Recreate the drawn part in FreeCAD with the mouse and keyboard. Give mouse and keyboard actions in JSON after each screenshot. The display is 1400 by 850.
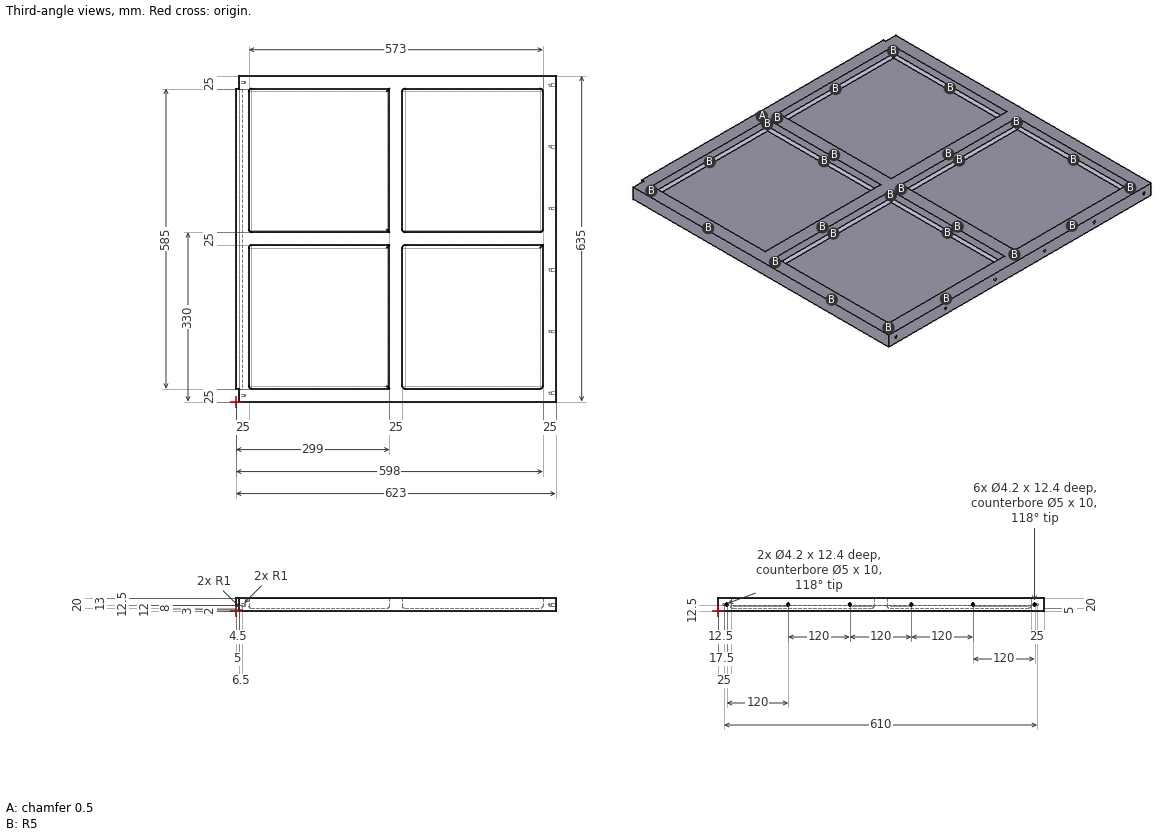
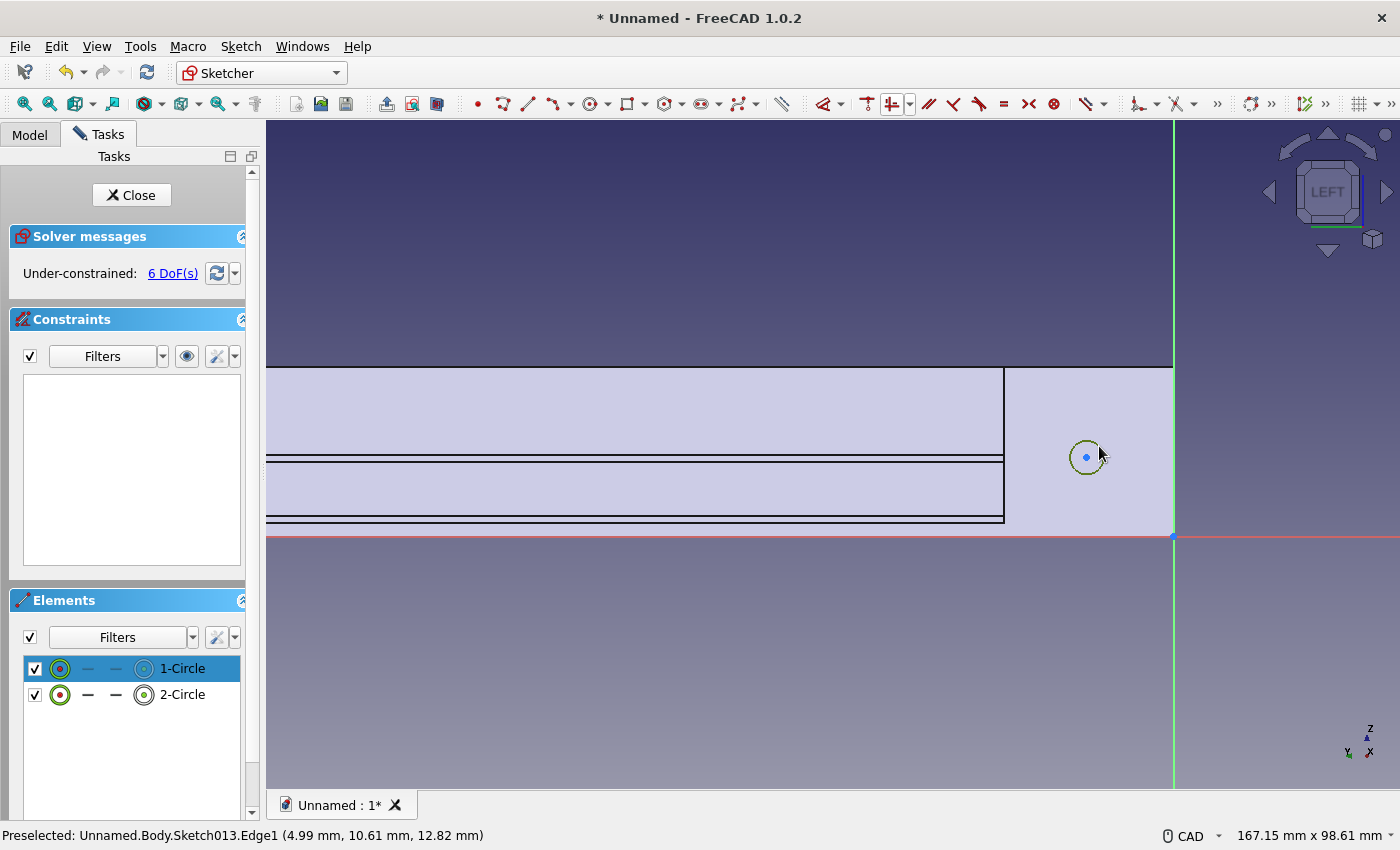
{"action": "scroll", "coordinate": [1103, 448], "scroll_direction": "down", "scroll_amount": 9}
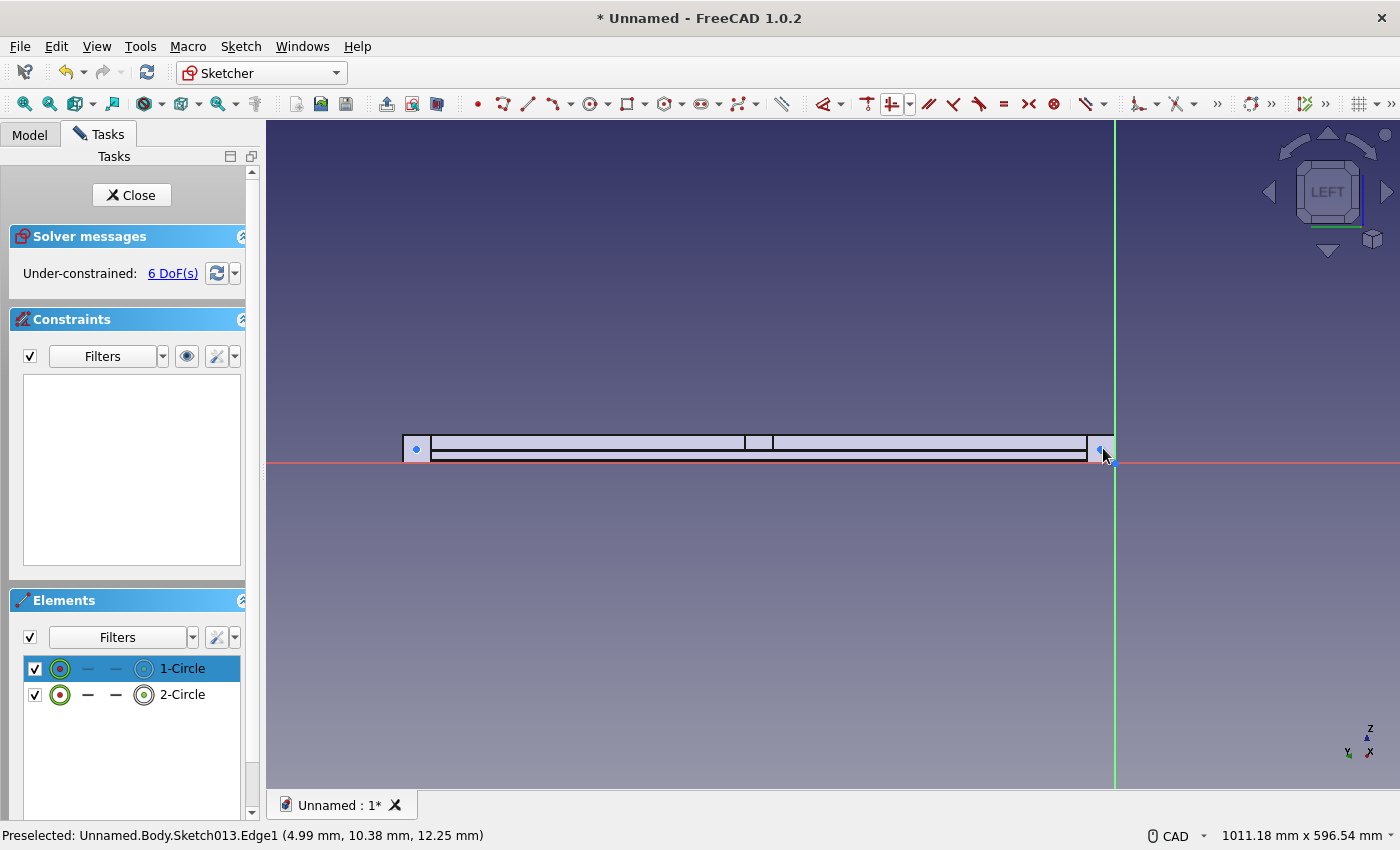
{"action": "scroll", "coordinate": [419, 448], "scroll_direction": "up", "scroll_amount": 8}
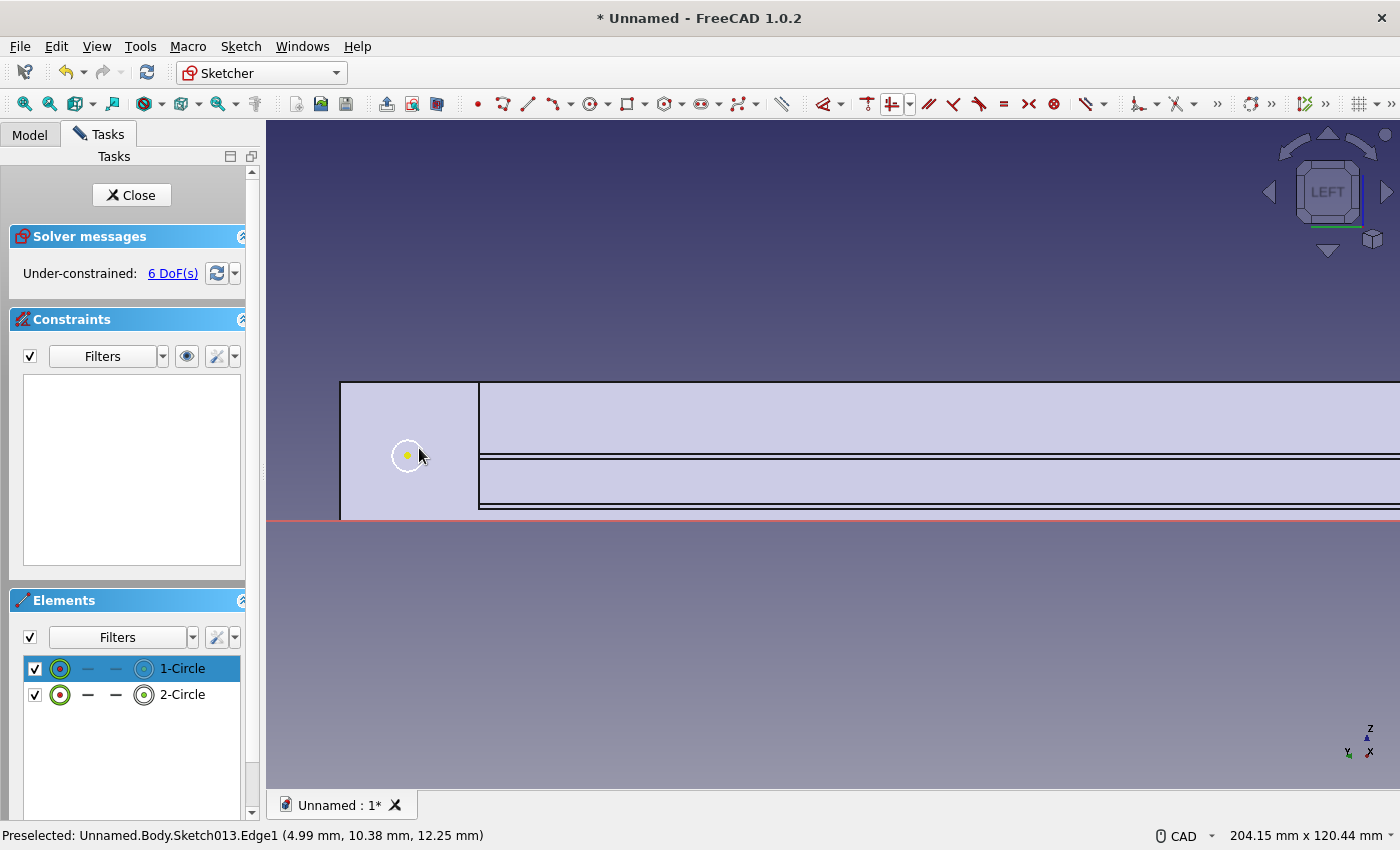
{"action": "left_click", "coordinate": [419, 445]}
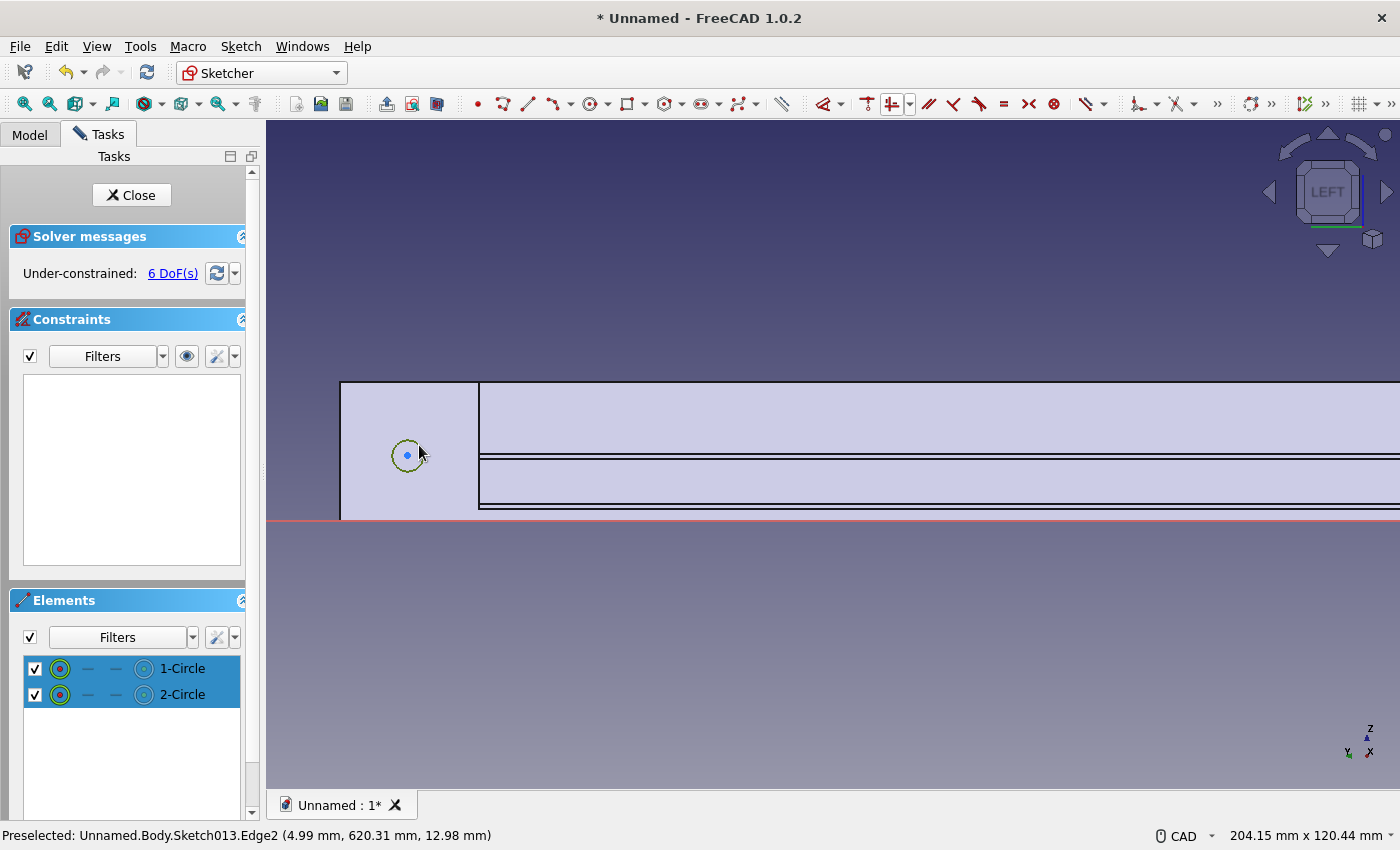
{"action": "left_click", "coordinate": [1004, 104]}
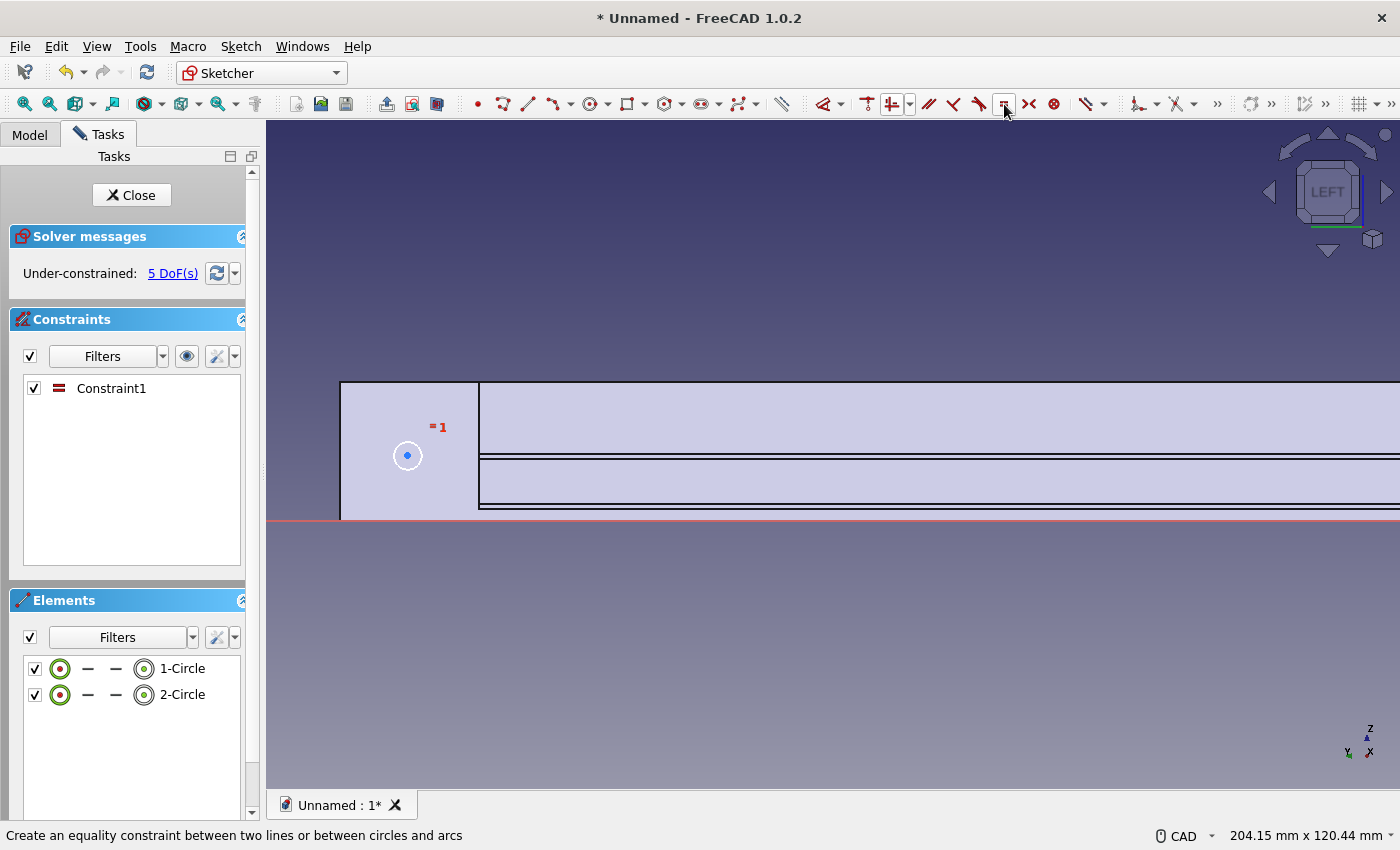
{"action": "left_click", "coordinate": [822, 104]}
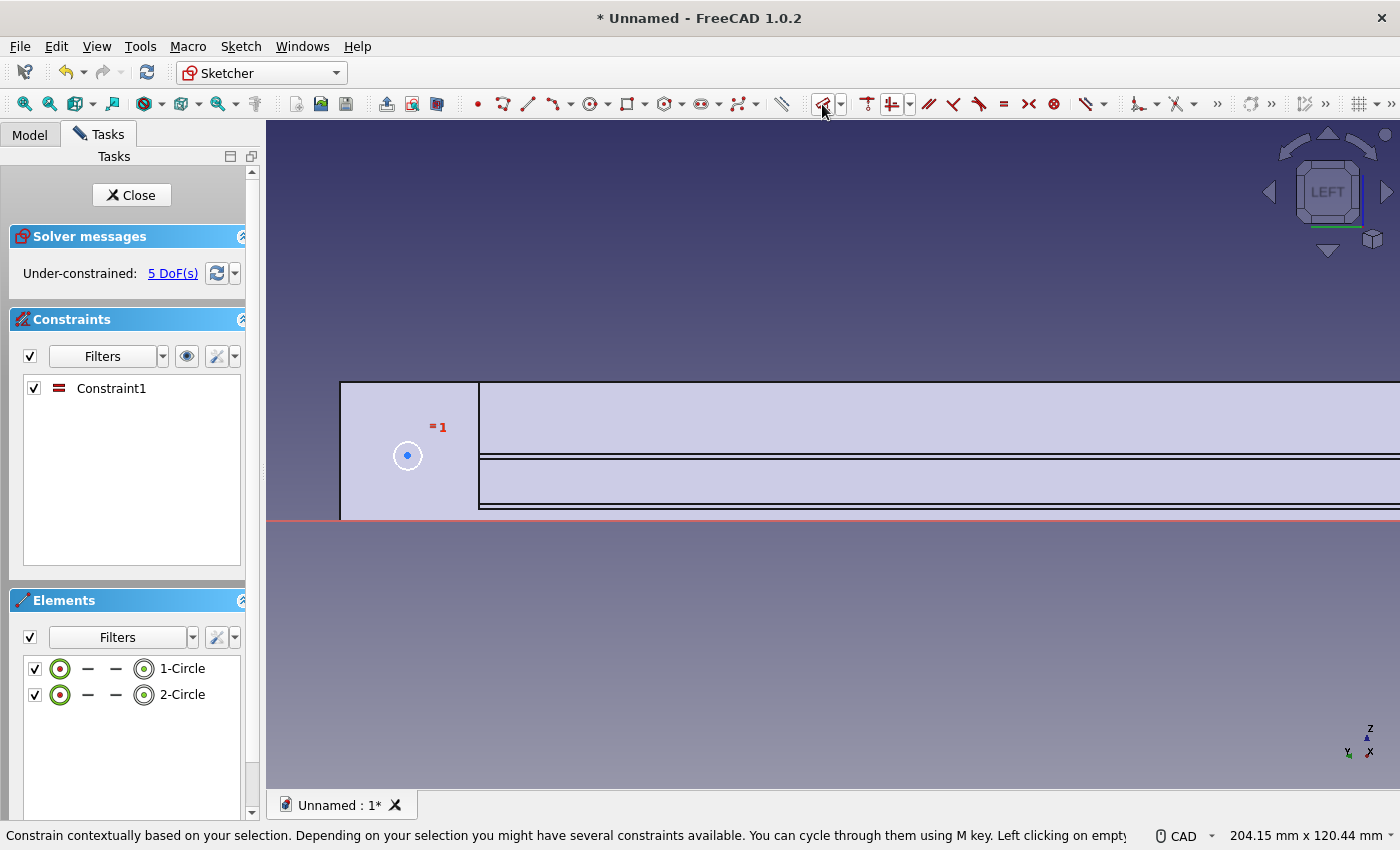
{"action": "scroll", "coordinate": [418, 448], "scroll_direction": "down", "scroll_amount": 8}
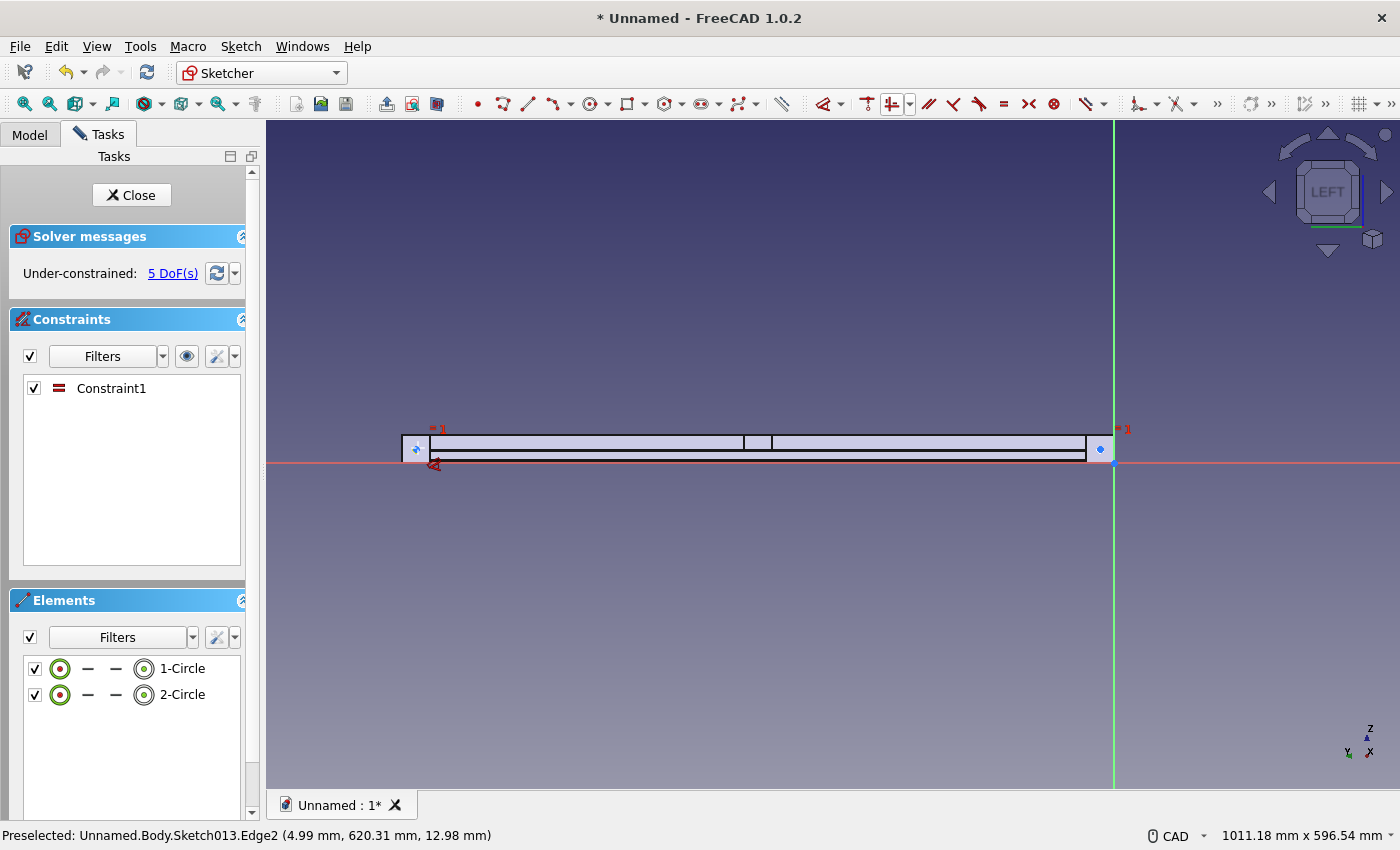
{"action": "scroll", "coordinate": [1102, 448], "scroll_direction": "up", "scroll_amount": 11}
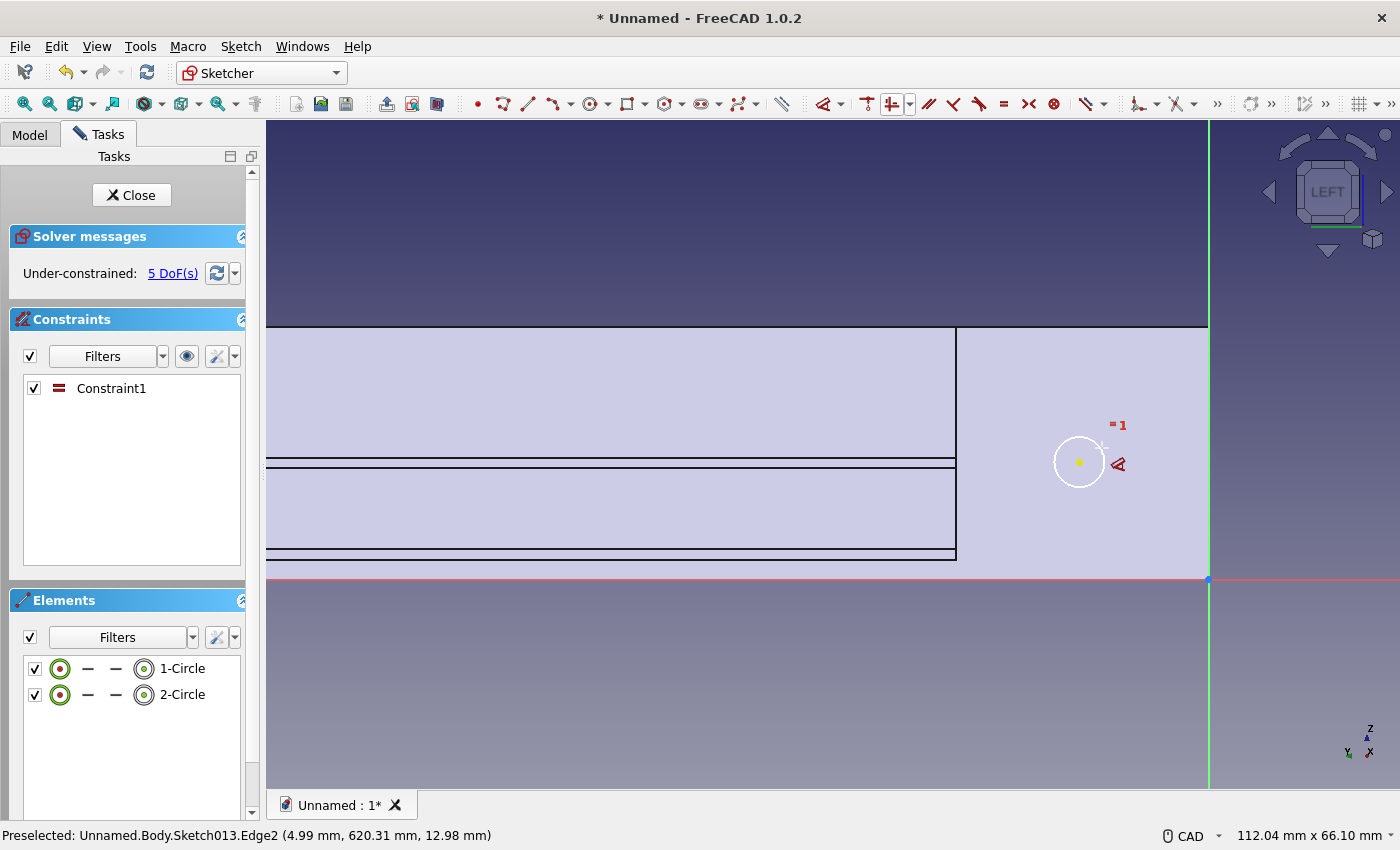
{"action": "left_click", "coordinate": [1097, 444]}
{"action": "left_click", "coordinate": [1119, 421]}